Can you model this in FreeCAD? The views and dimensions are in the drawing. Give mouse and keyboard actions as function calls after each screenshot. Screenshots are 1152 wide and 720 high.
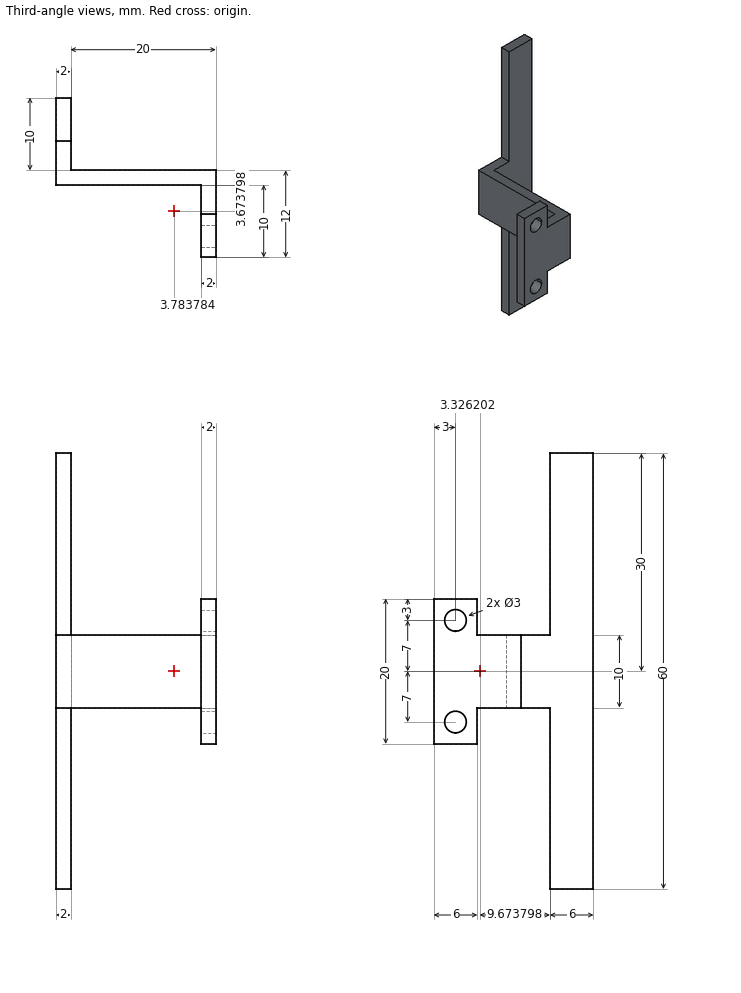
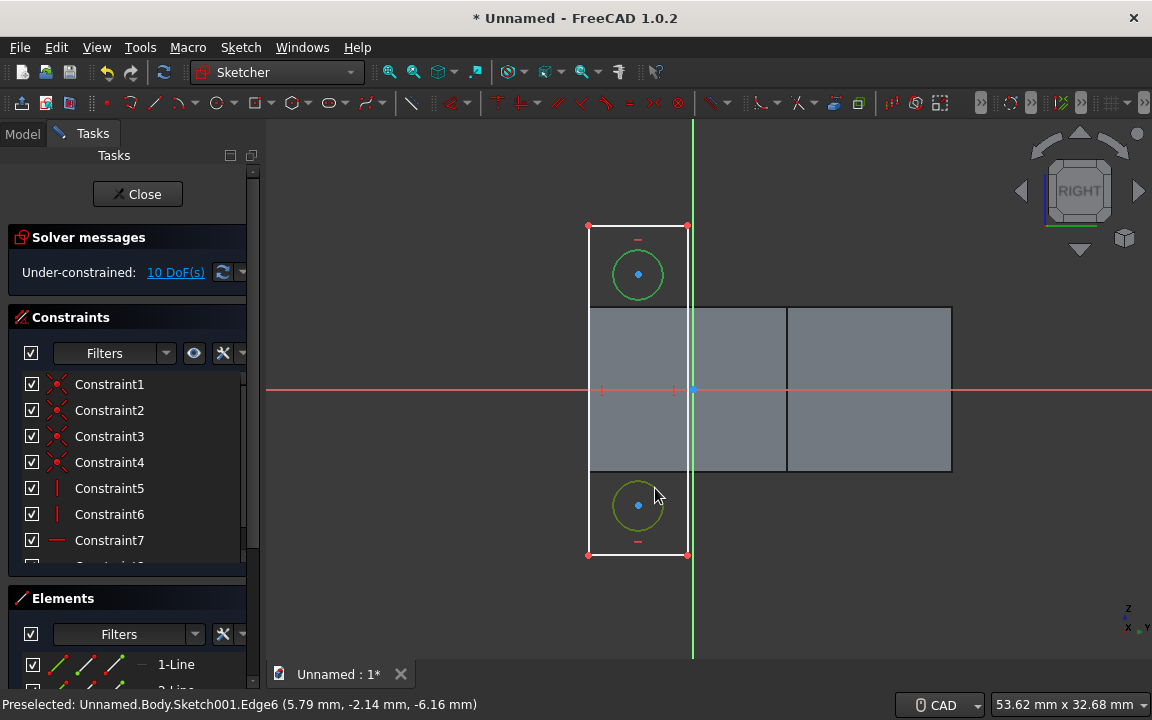
key(e)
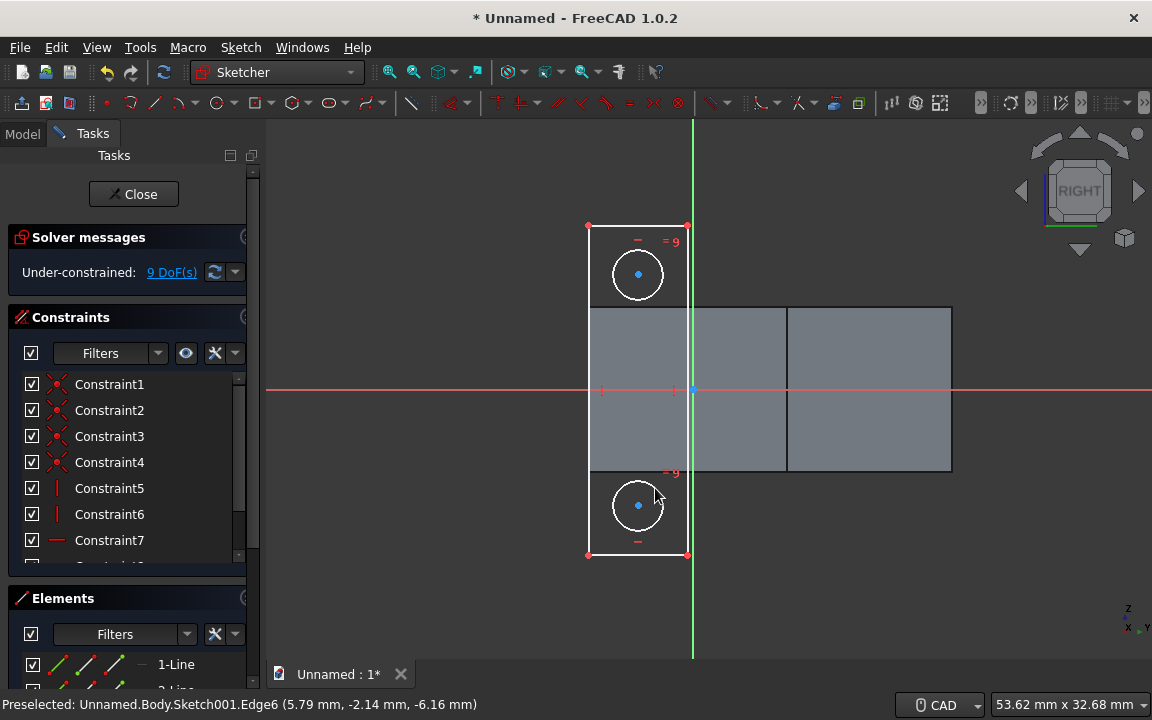
key(d)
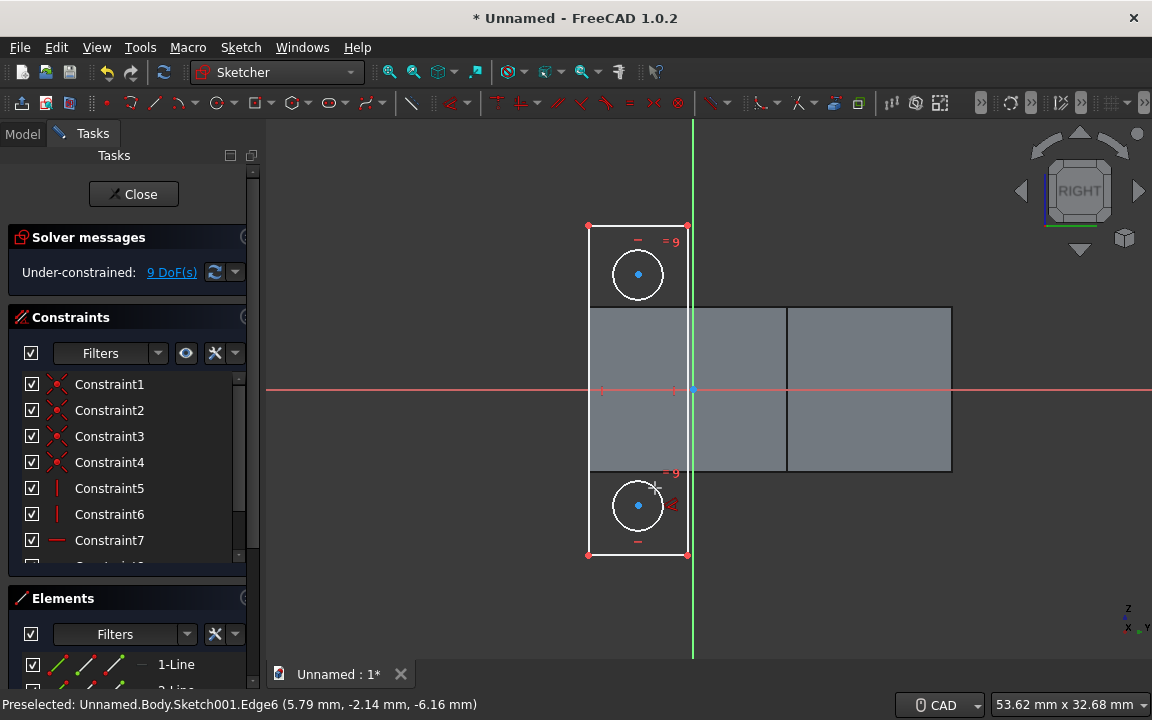
click(655, 257)
click(714, 250)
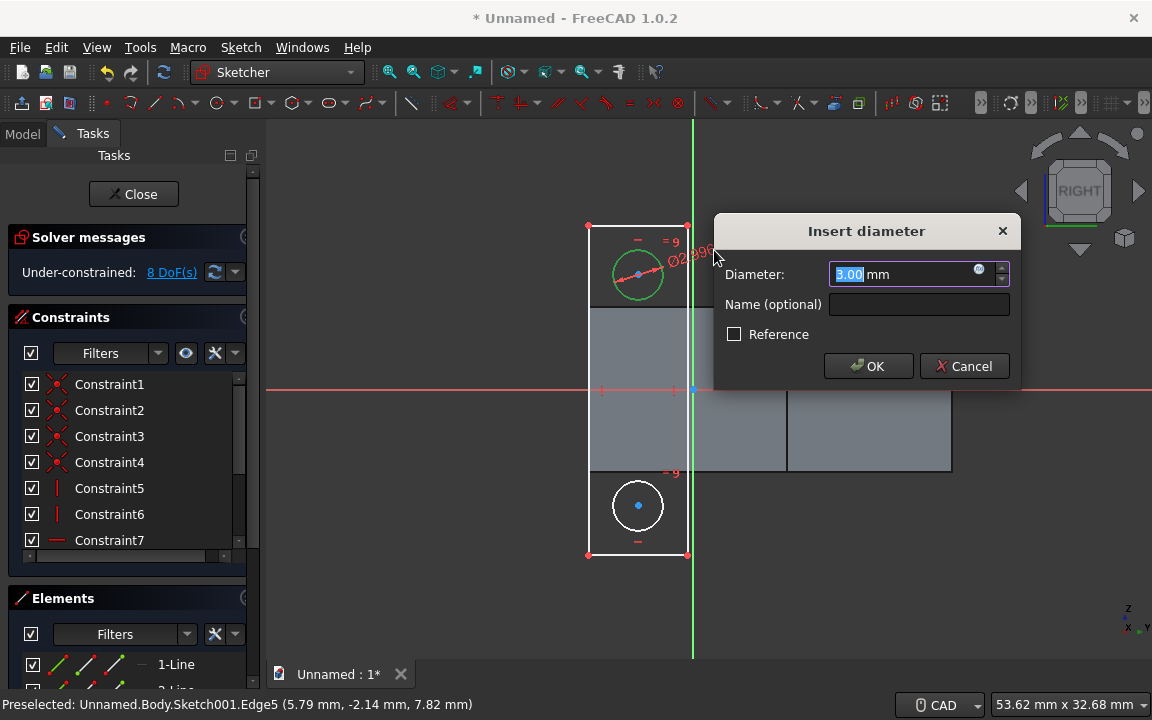
text(3)
key(Return)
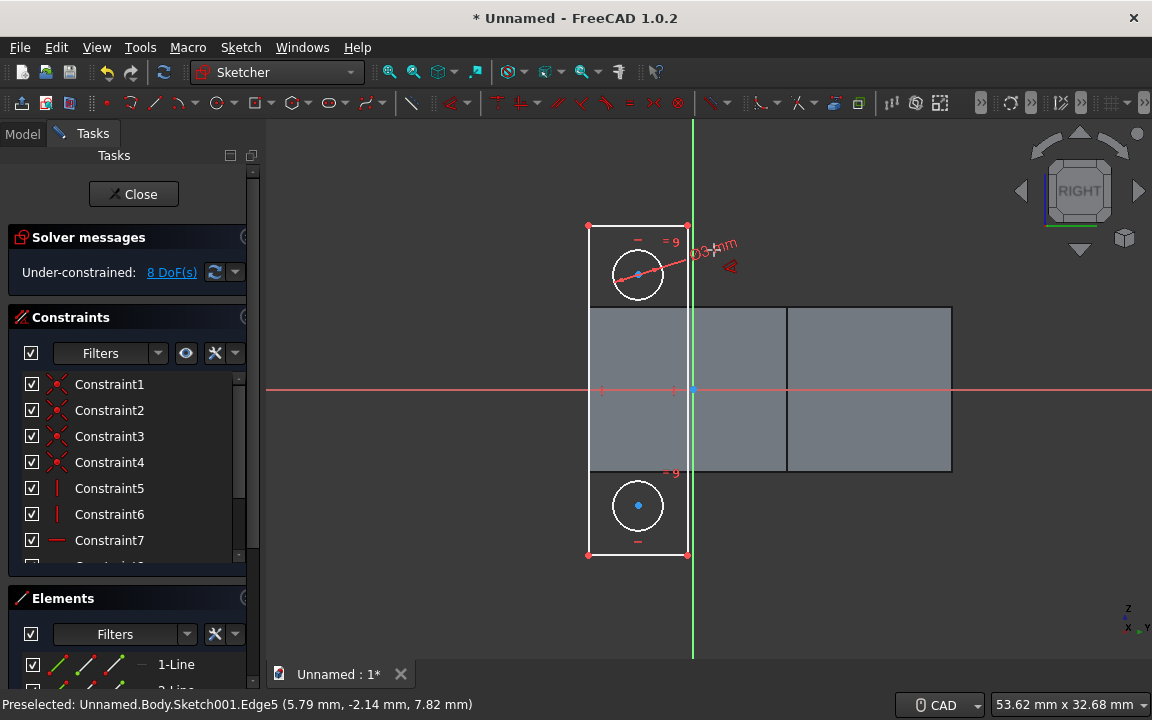
click(618, 555)
click(638, 589)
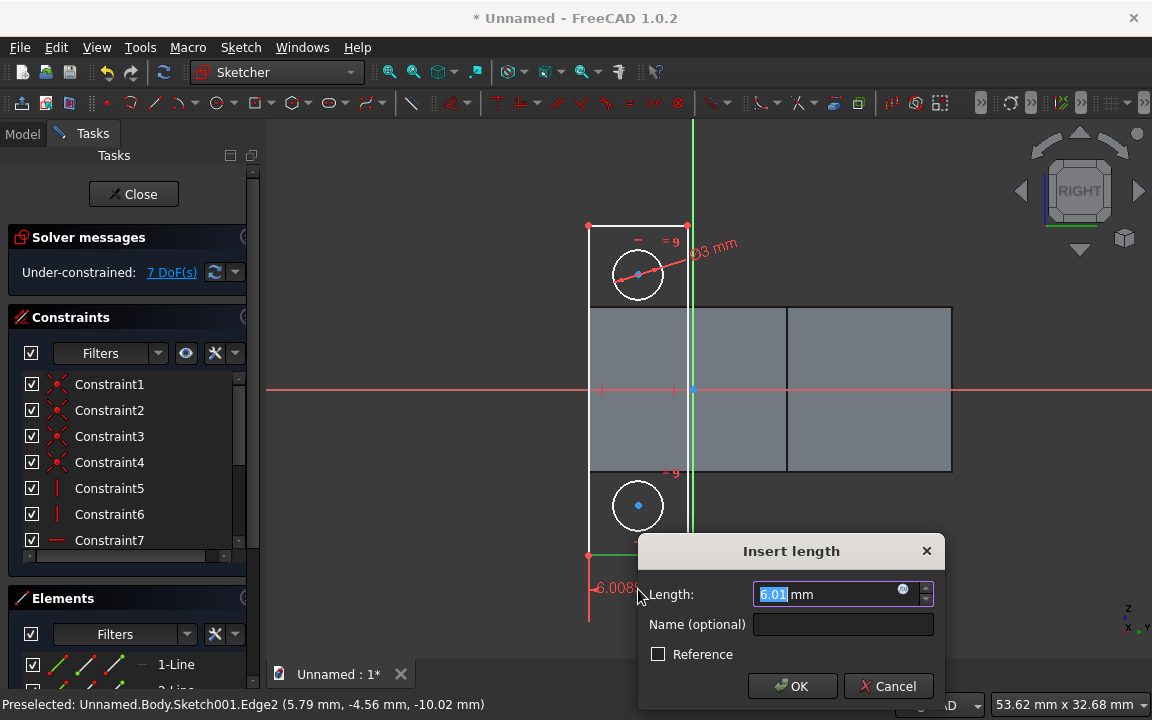
text(6)
key(Return)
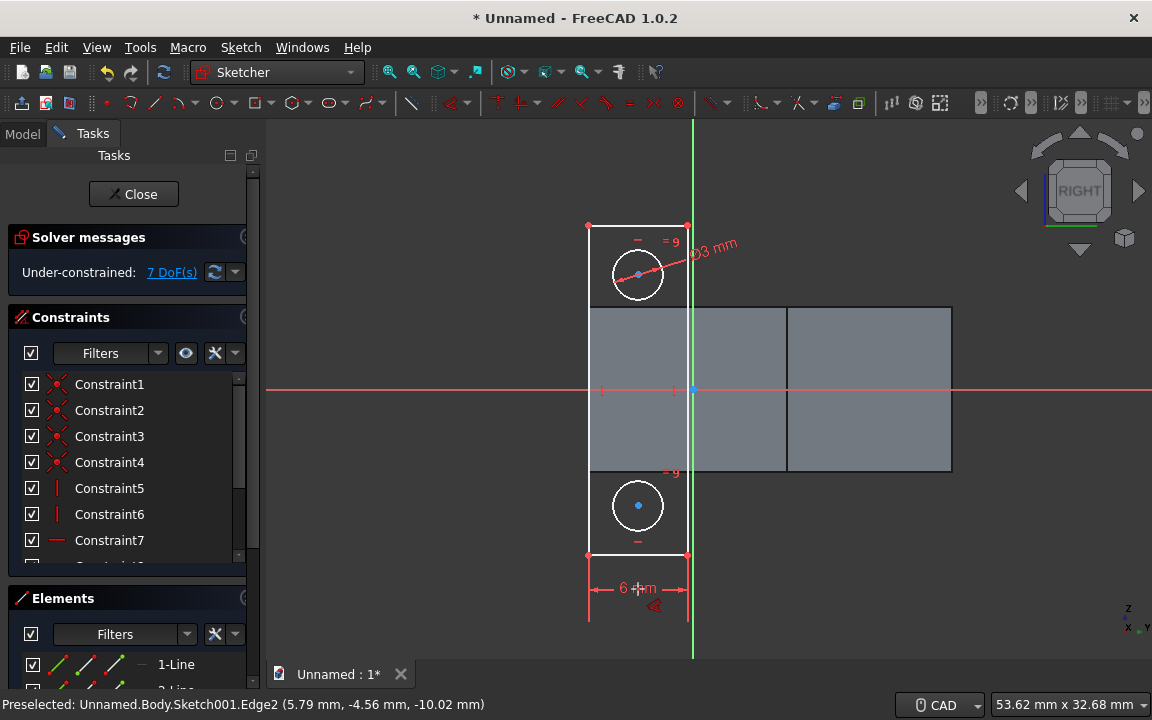
click(638, 275)
click(727, 332)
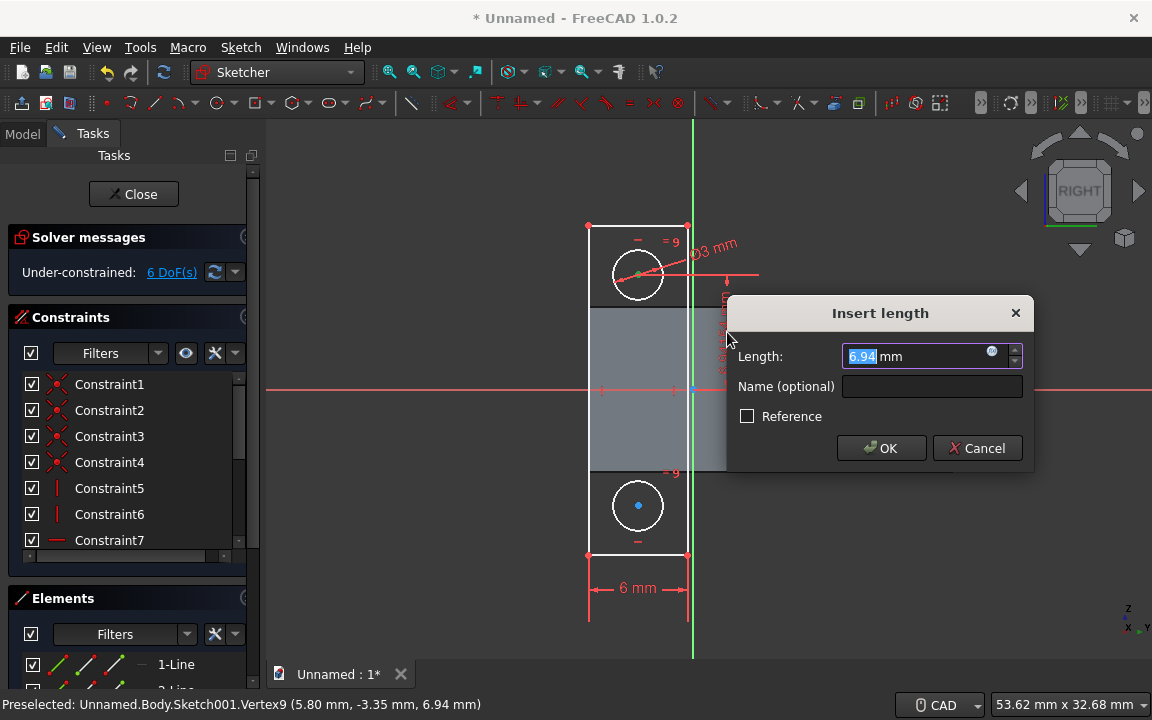
text(7)
key(Return)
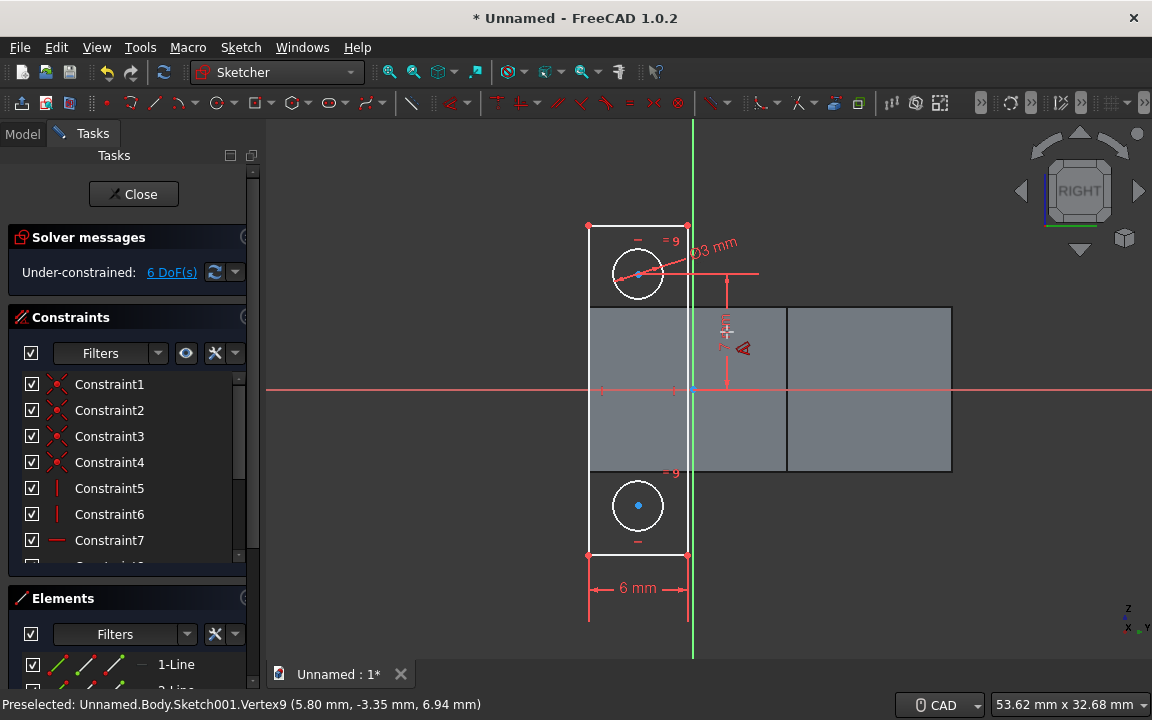
click(638, 506)
click(727, 448)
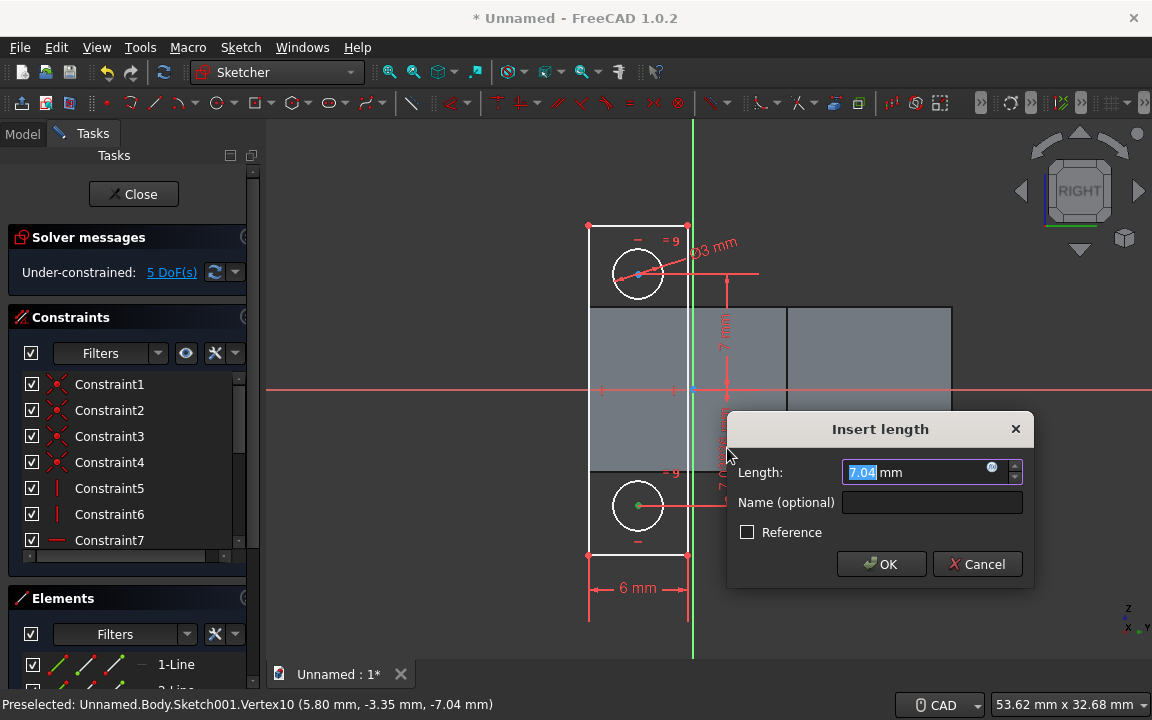
text(7)
key(Return)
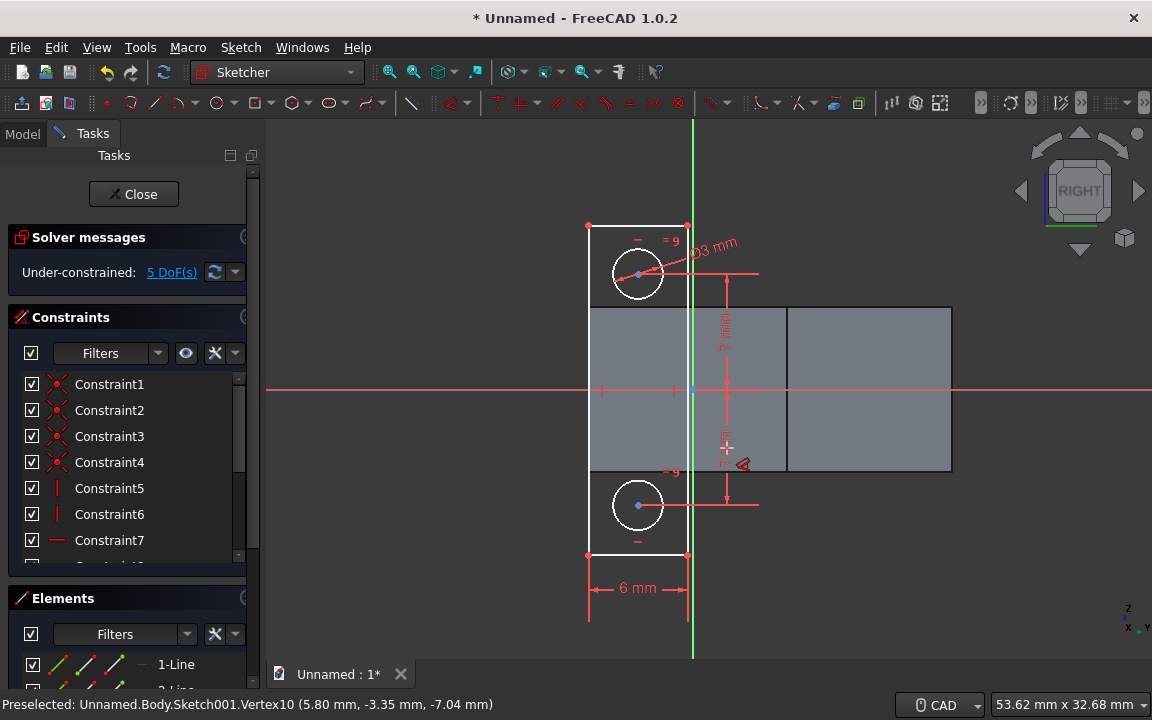
click(589, 325)
click(555, 315)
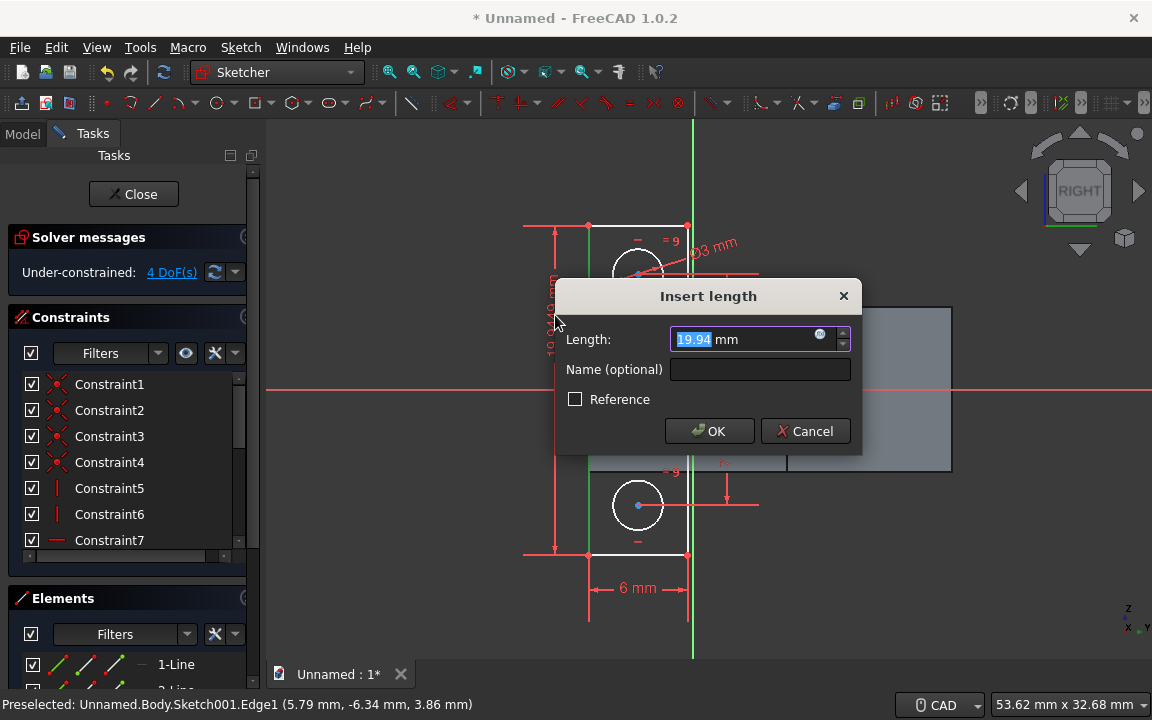
text(20)
key(Return)